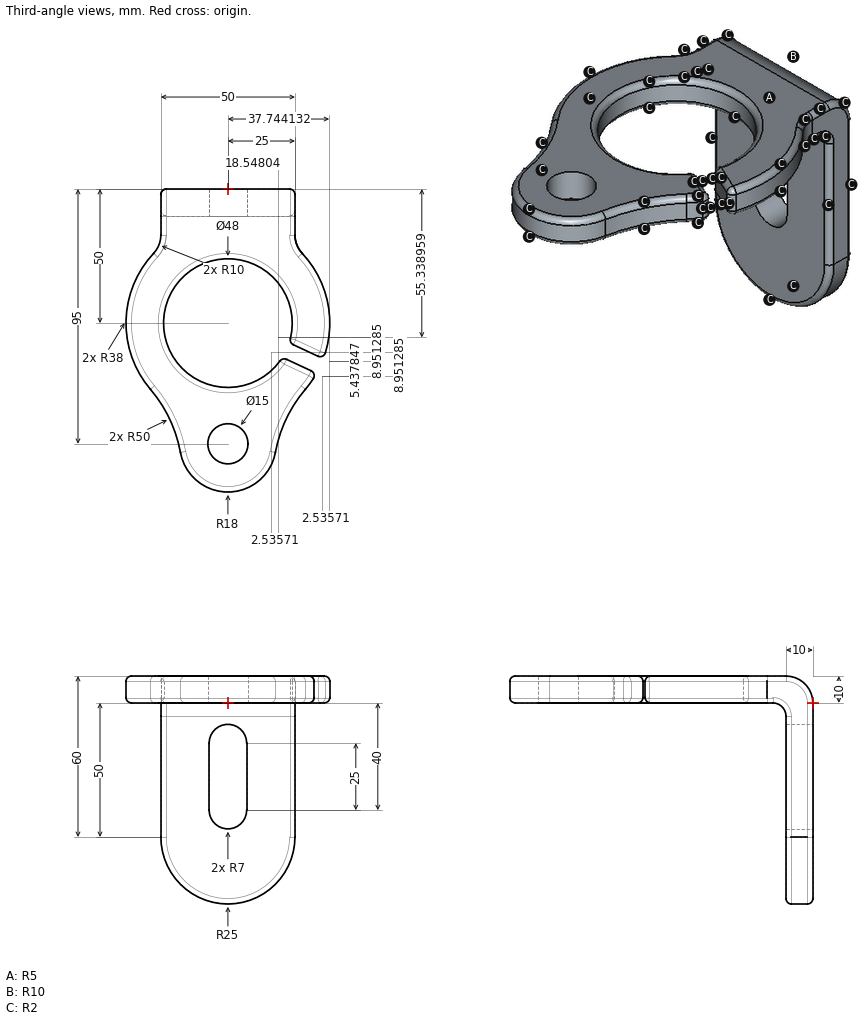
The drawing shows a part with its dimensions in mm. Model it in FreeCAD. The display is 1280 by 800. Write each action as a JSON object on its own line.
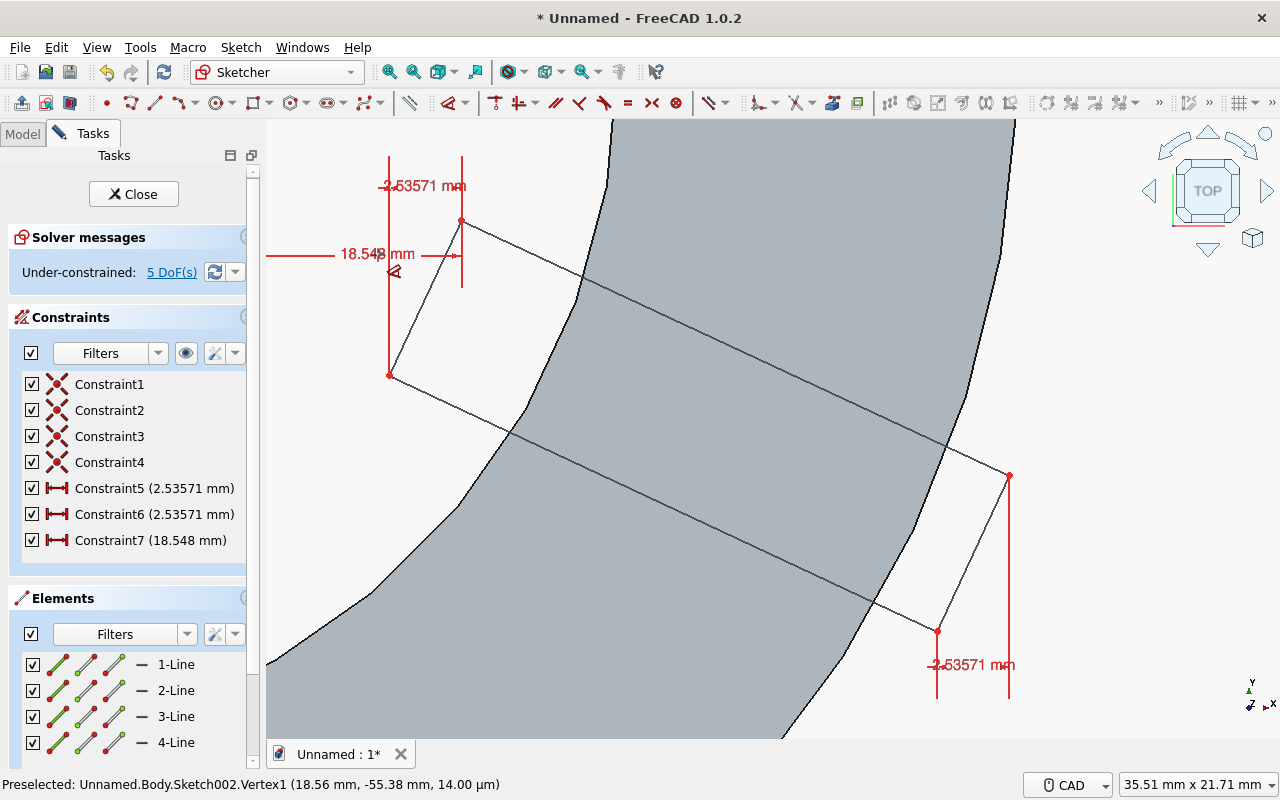
{"action": "left_click", "coordinate": [626, 297]}
{"action": "left_click", "coordinate": [1043, 348]}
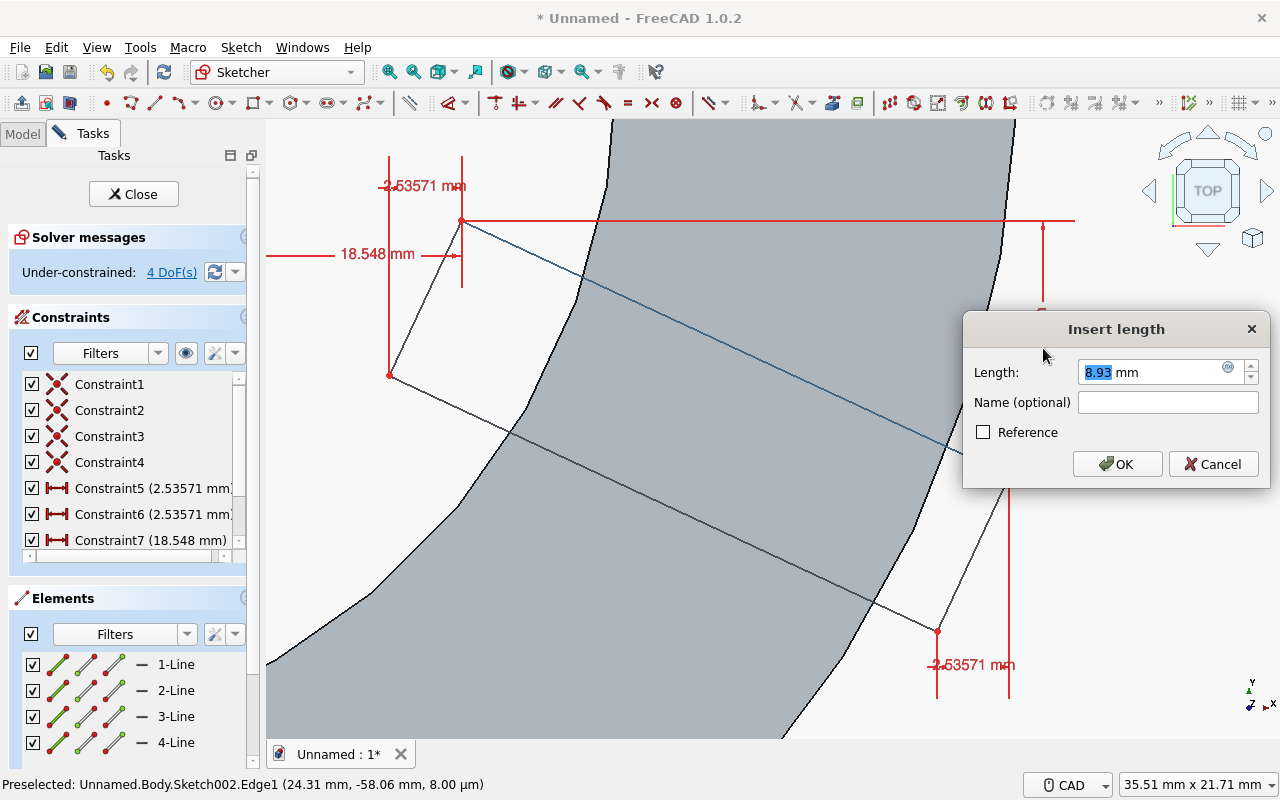
{"action": "type", "text": "8.951285"}
{"action": "key", "text": "Return"}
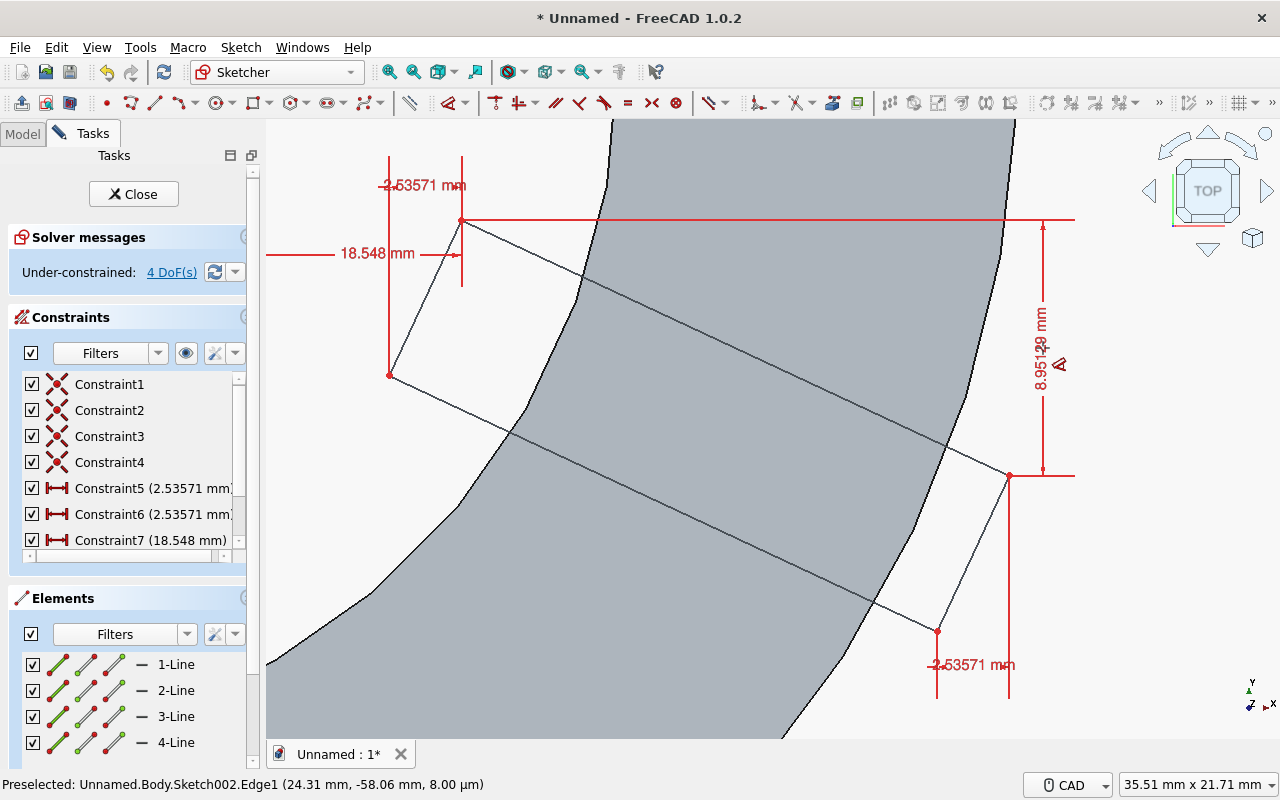
{"action": "left_click", "coordinate": [988, 523]}
{"action": "left_click", "coordinate": [1043, 554]}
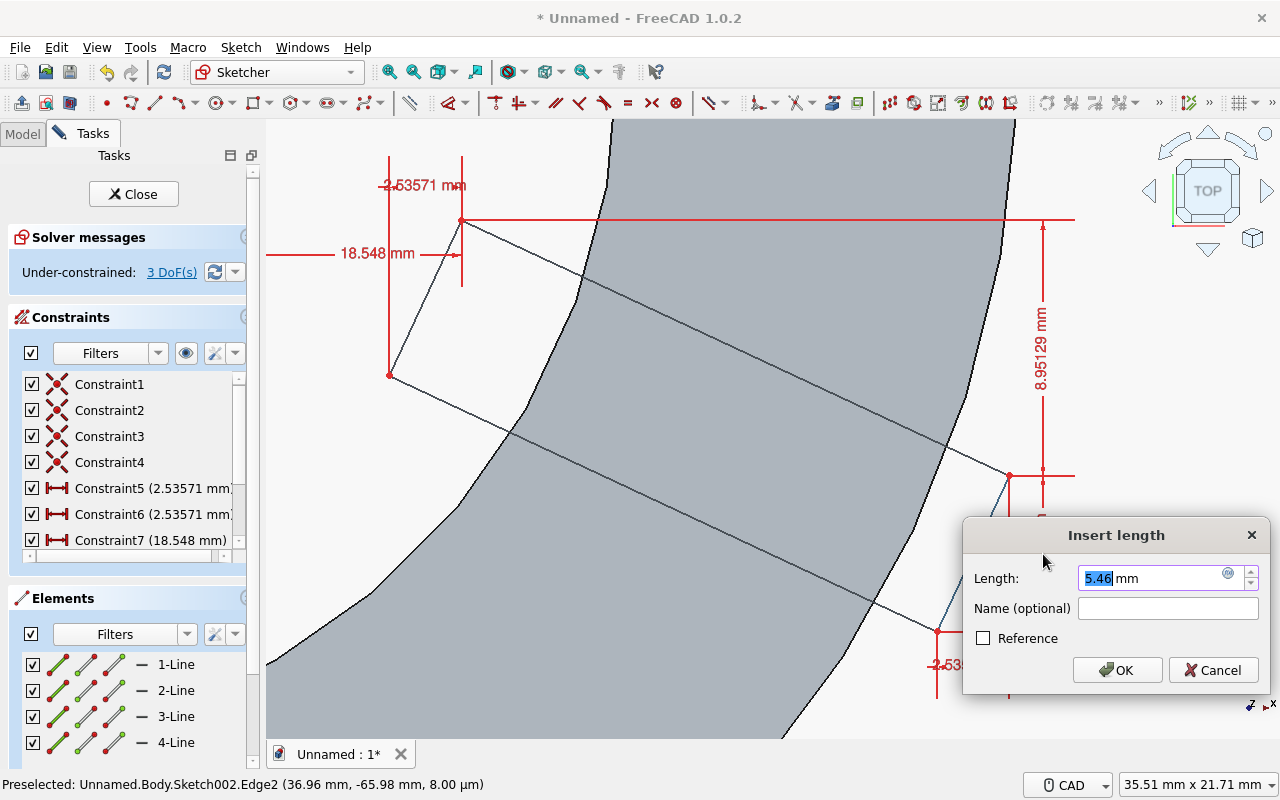
{"action": "type", "text": "5.437847"}
{"action": "key", "text": "Return"}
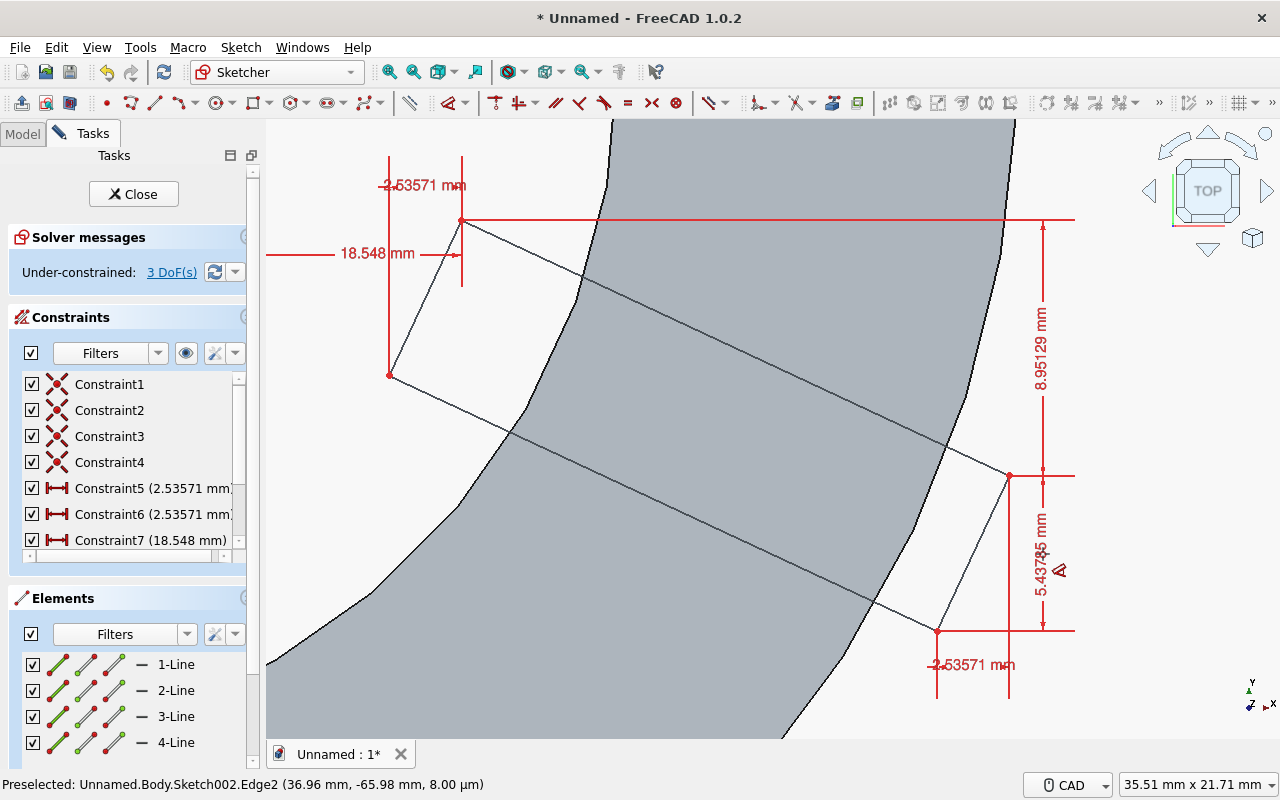
{"action": "left_click", "coordinate": [773, 555]}
{"action": "left_click", "coordinate": [355, 504]}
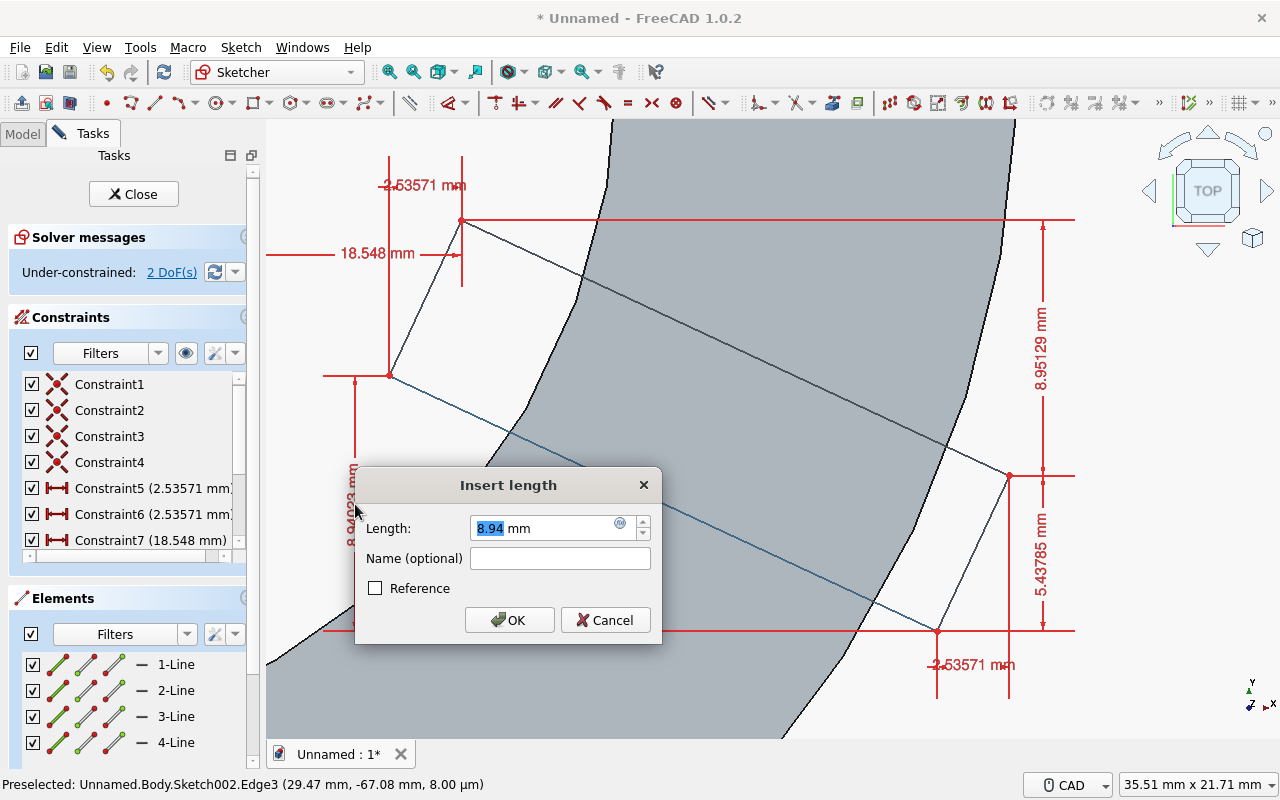
{"action": "type", "text": "8.951285"}
{"action": "key", "text": "Return"}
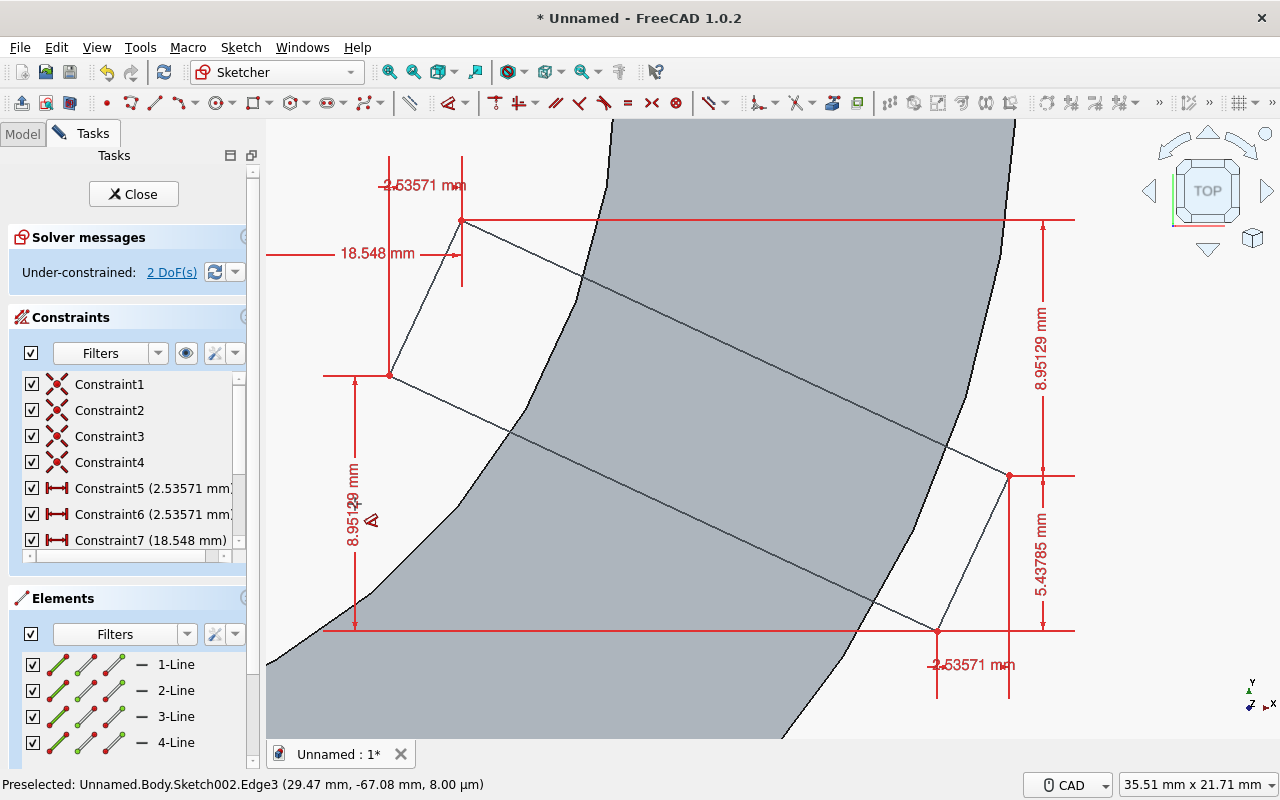
{"action": "left_click", "coordinate": [462, 220]}
{"action": "left_click", "coordinate": [496, 184]}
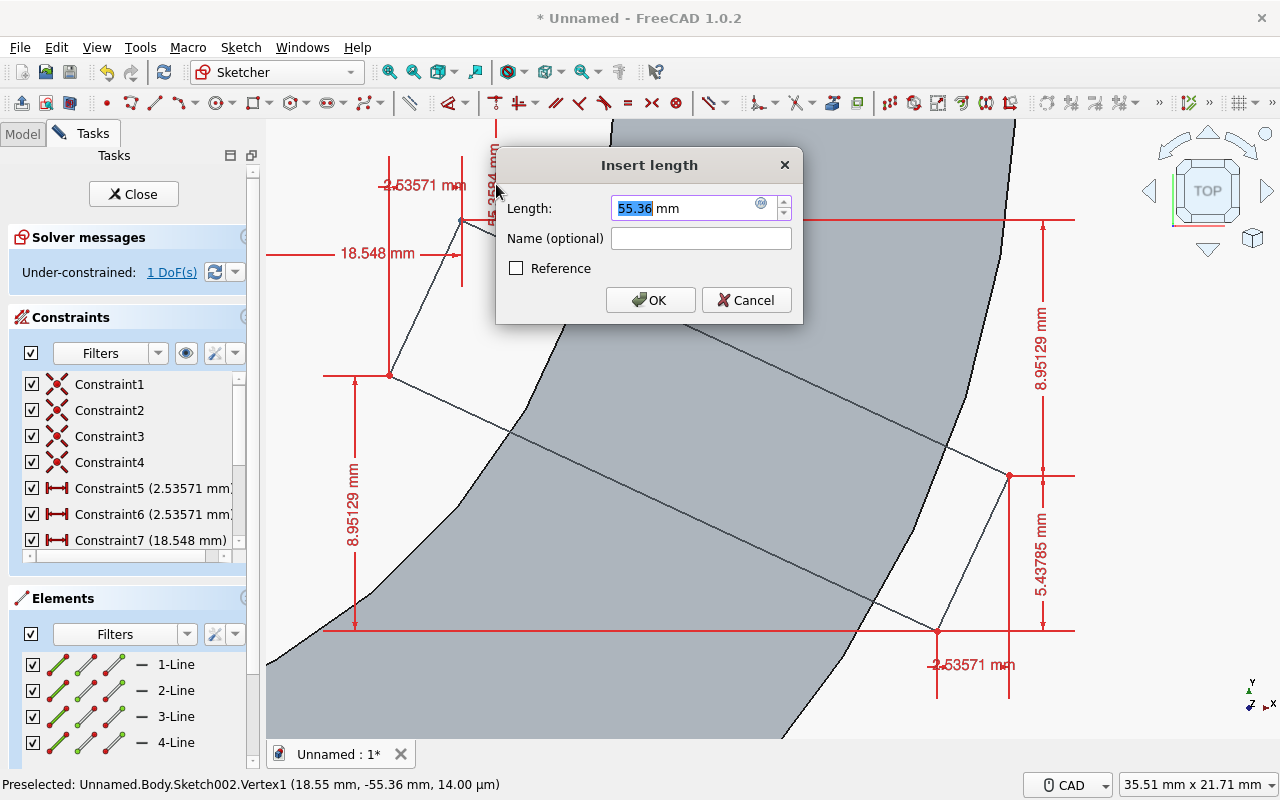
{"action": "type", "text": "55.338959"}
{"action": "key", "text": "Return"}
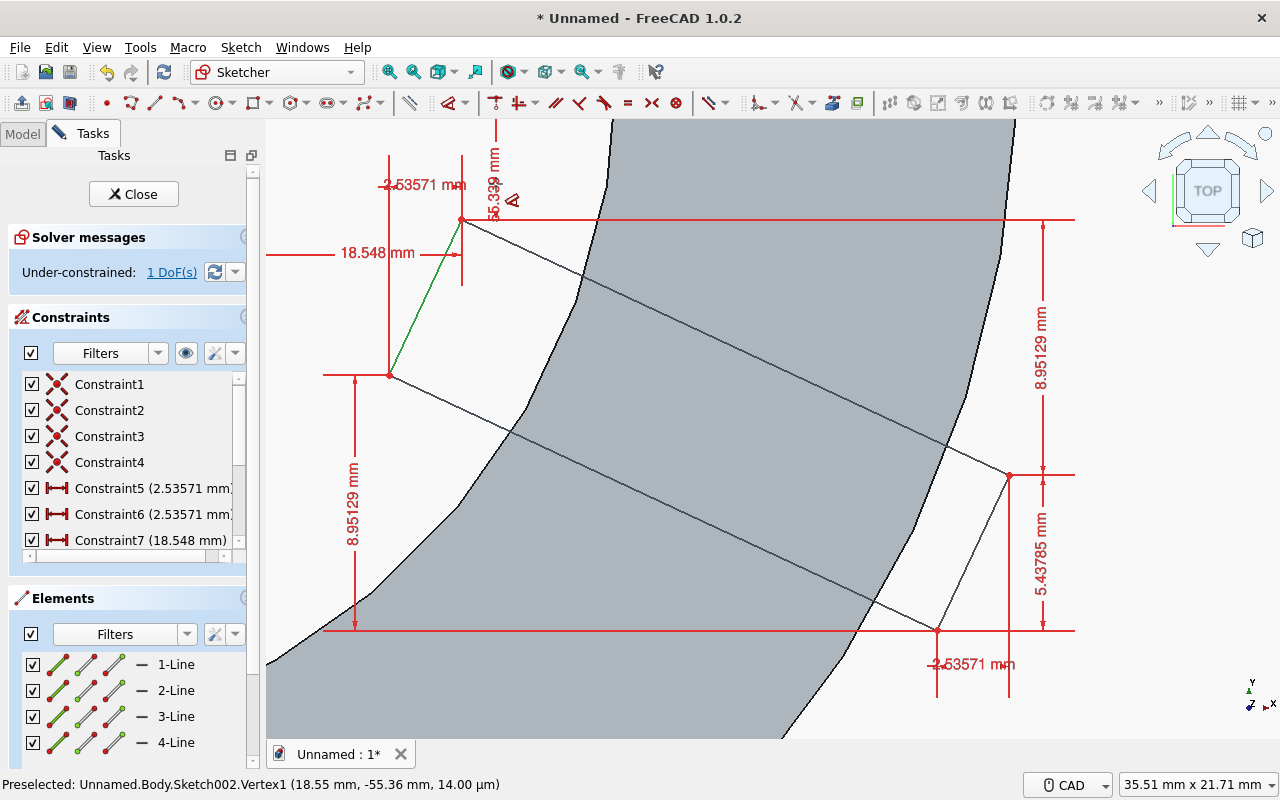
{"action": "left_click", "coordinate": [1009, 475]}
{"action": "left_click", "coordinate": [487, 509]}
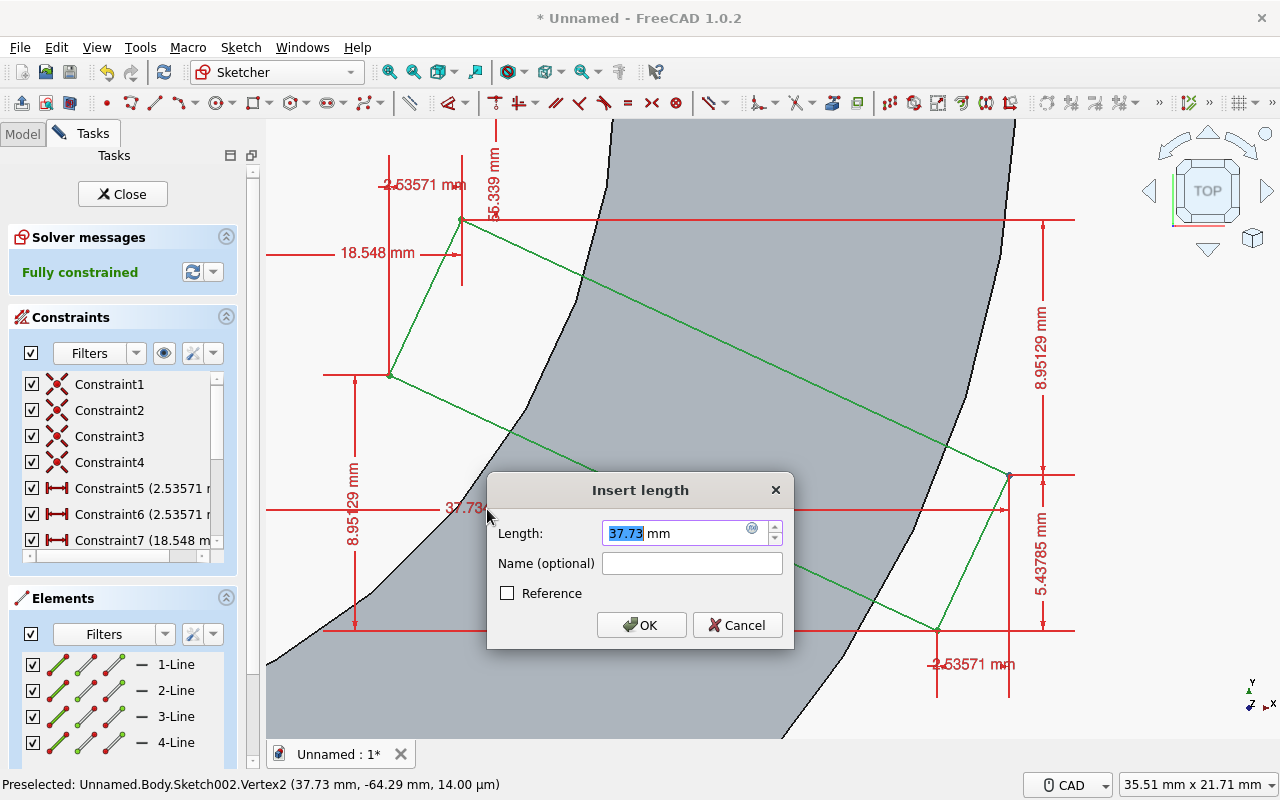
{"action": "type", "text": "37.744132"}
{"action": "key", "text": "Return"}
{"action": "key", "text": "Escape"}